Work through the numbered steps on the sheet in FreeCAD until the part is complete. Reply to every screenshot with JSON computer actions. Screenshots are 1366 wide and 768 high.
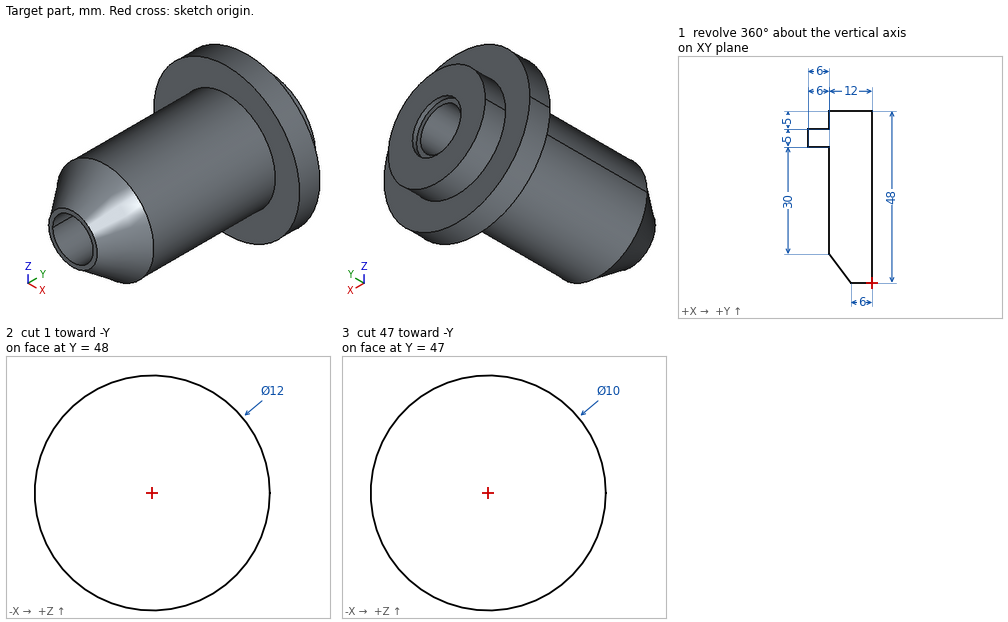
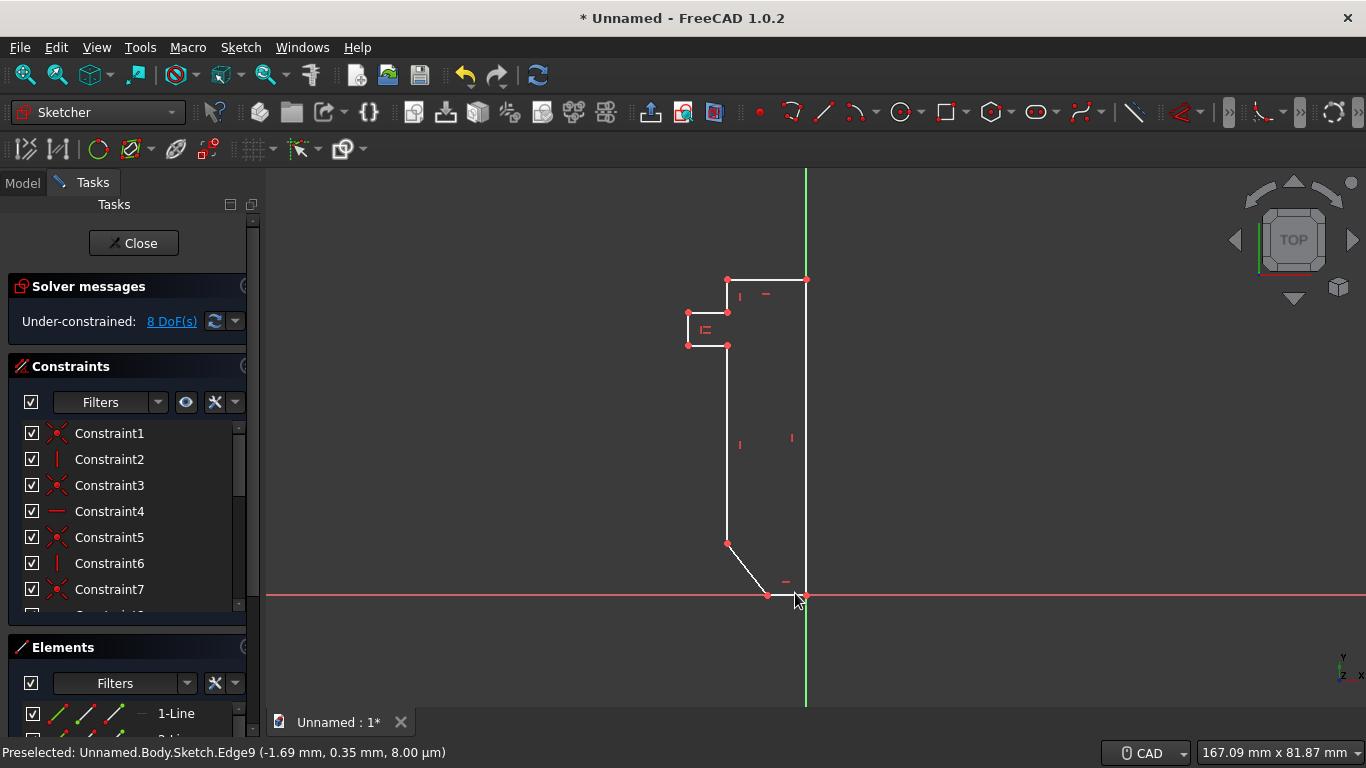
{"action": "scroll", "coordinate": [727, 290], "scroll_direction": "up", "scroll_amount": 2}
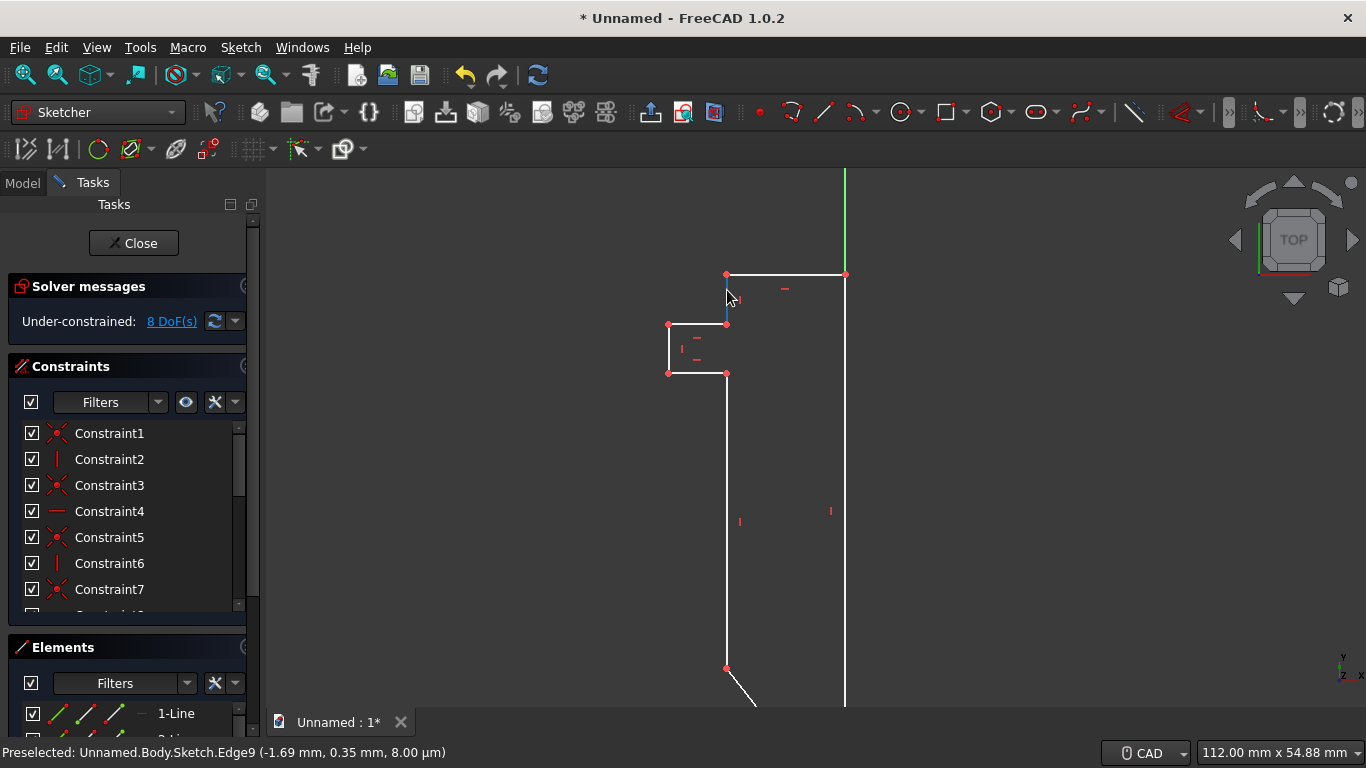
{"action": "left_click", "coordinate": [727, 290]}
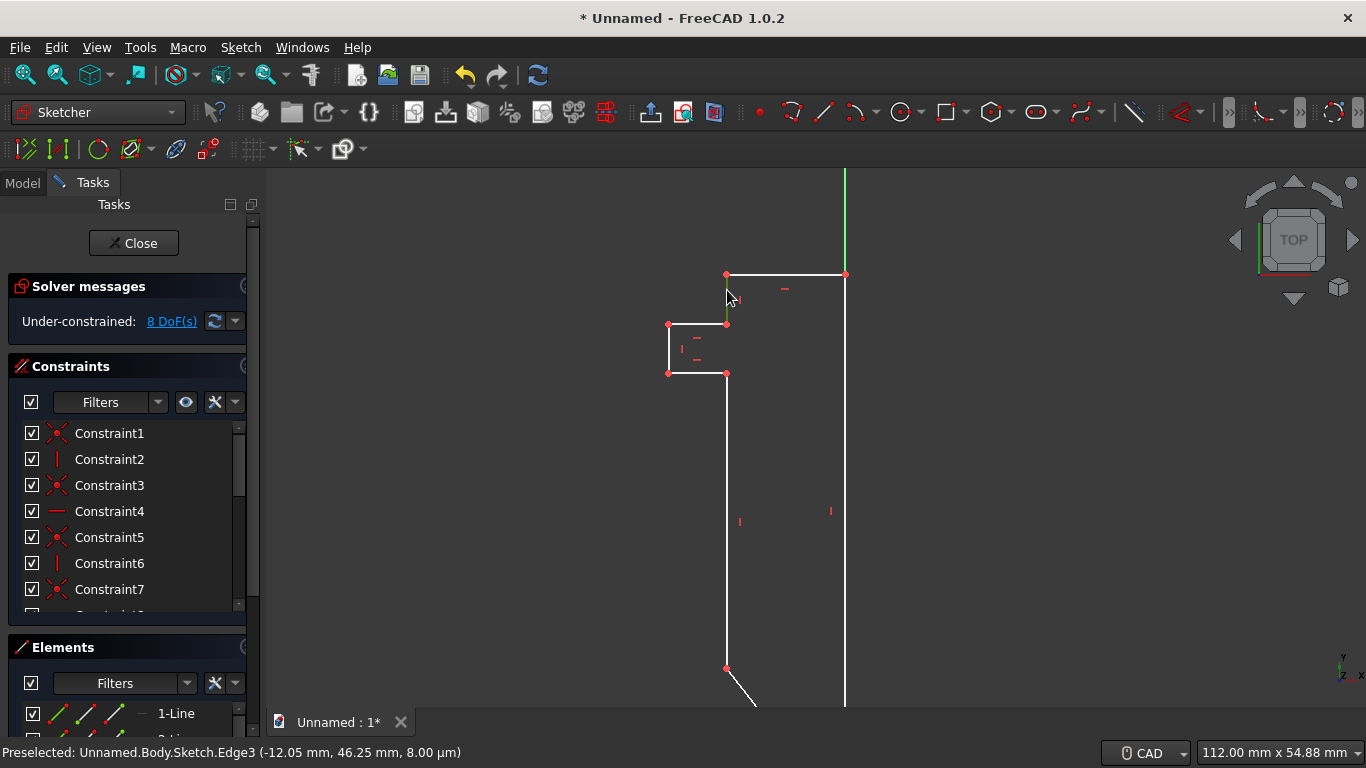
{"action": "left_click", "coordinate": [1202, 112]}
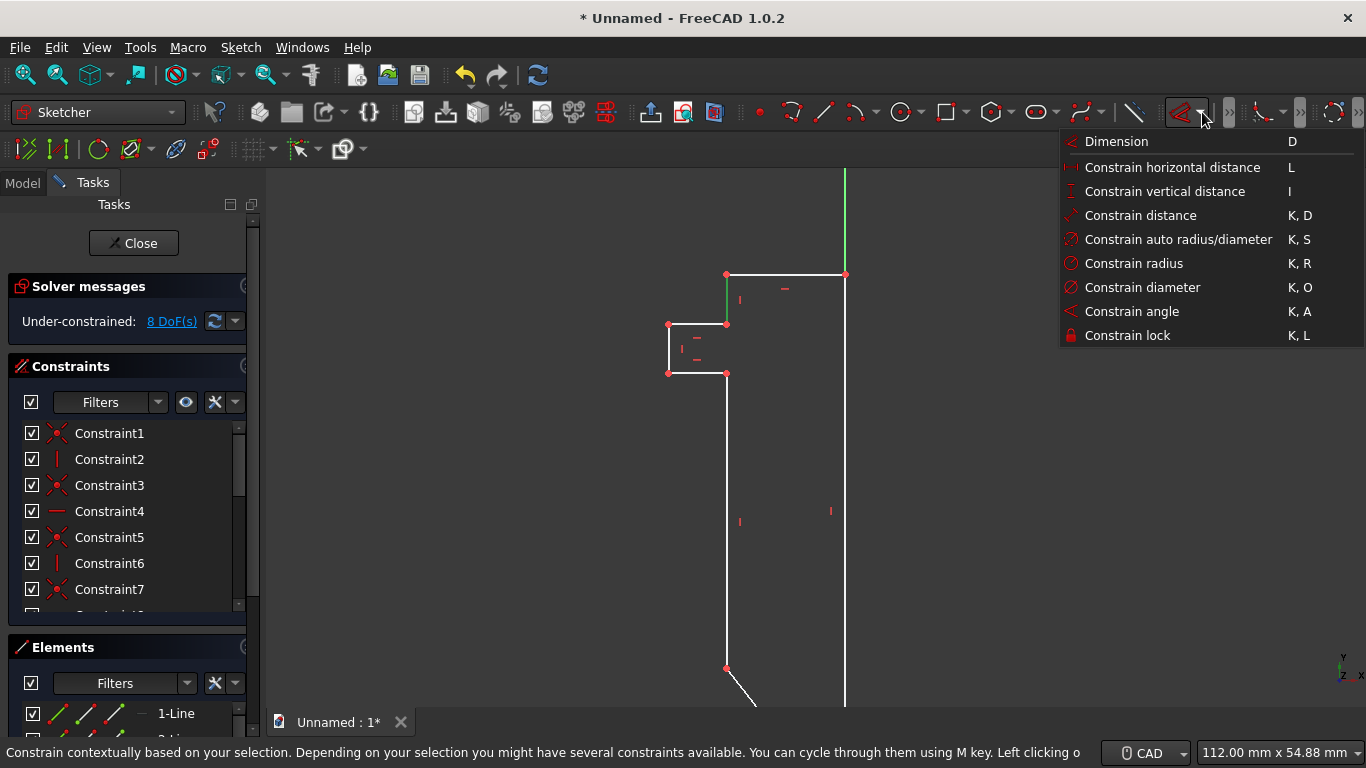
{"action": "left_click", "coordinate": [1212, 191]}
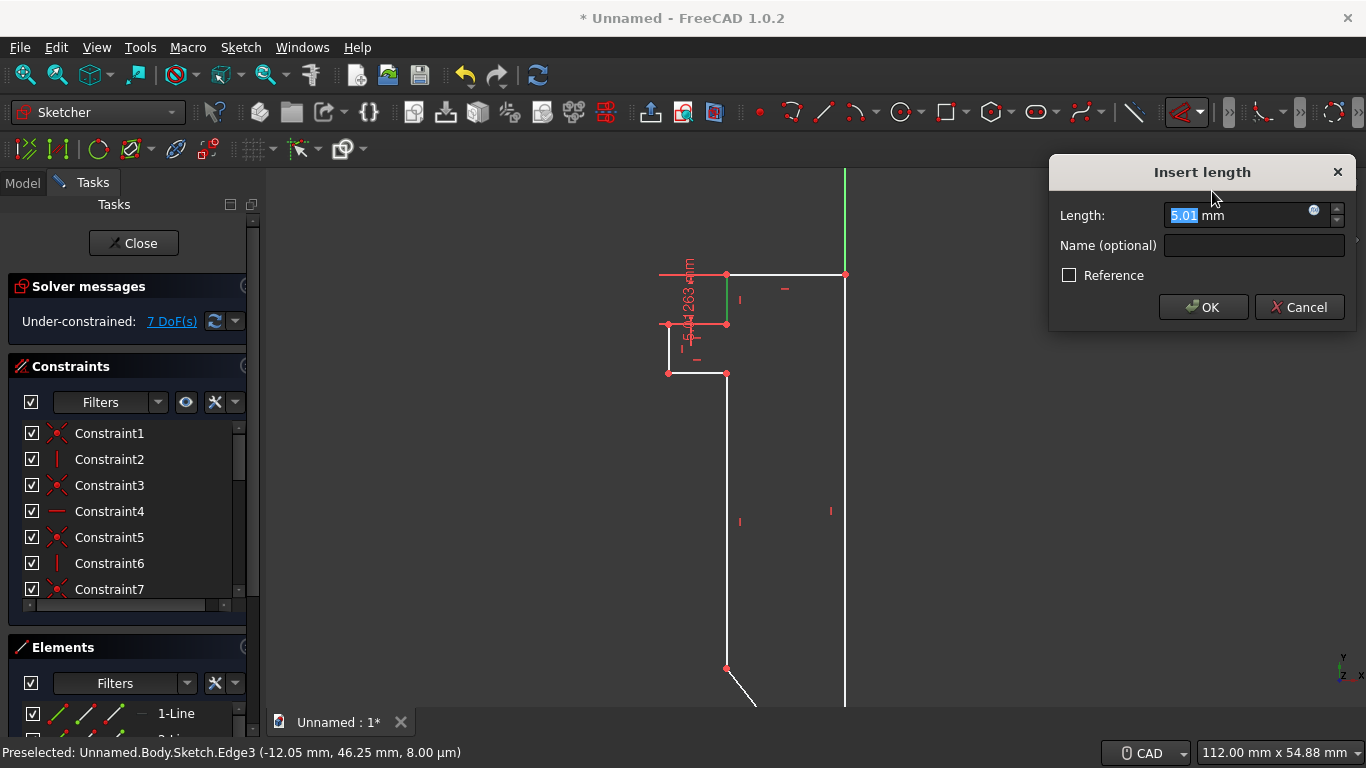
{"action": "type", "text": "5"}
{"action": "key", "text": "Return"}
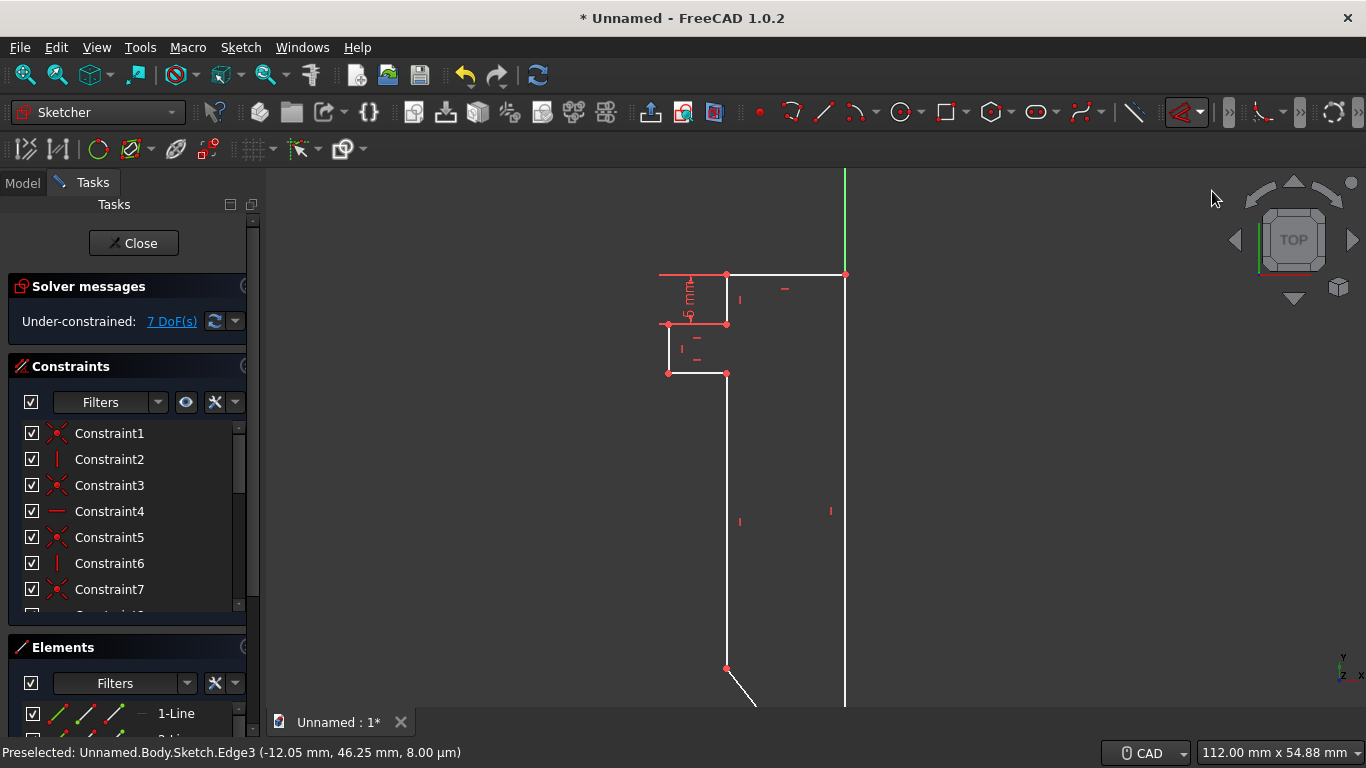
{"action": "left_click", "coordinate": [709, 324]}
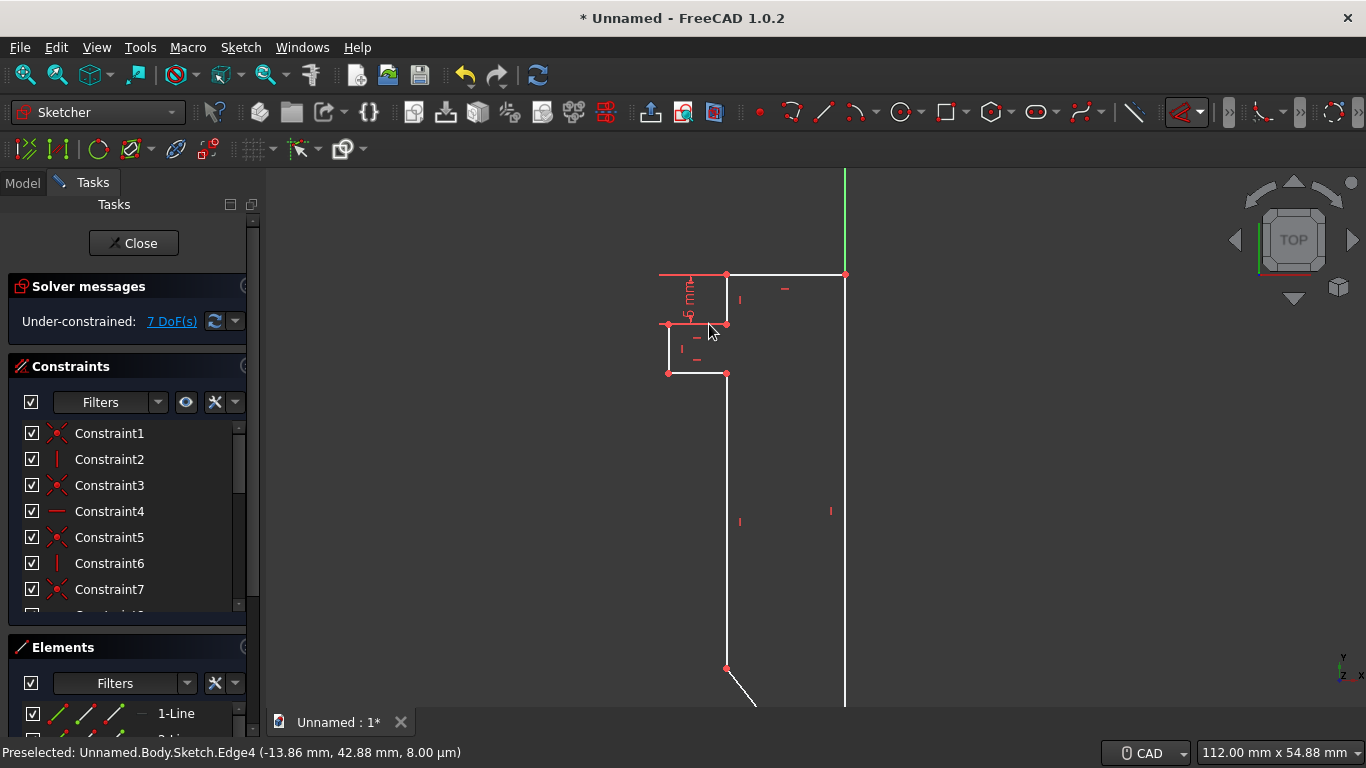
{"action": "left_click", "coordinate": [1202, 112]}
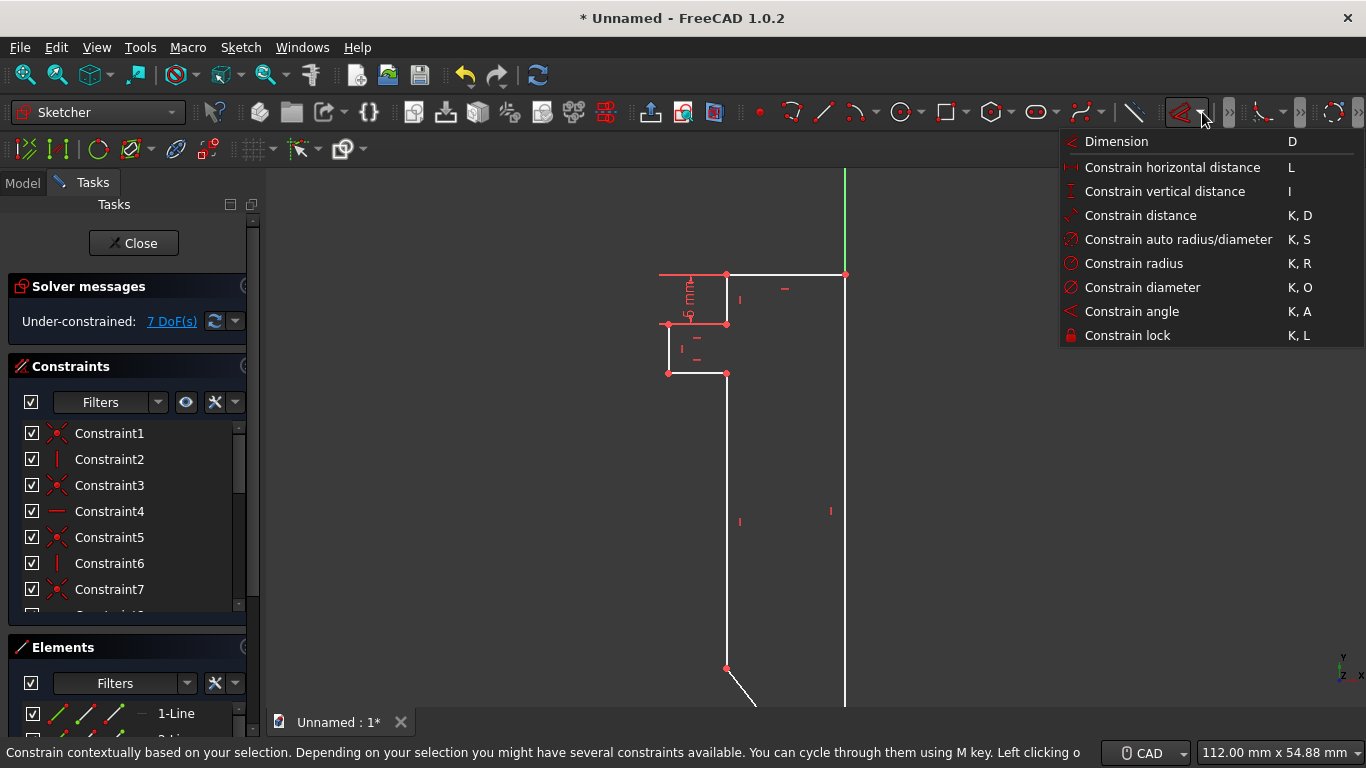
{"action": "left_click", "coordinate": [1212, 167]}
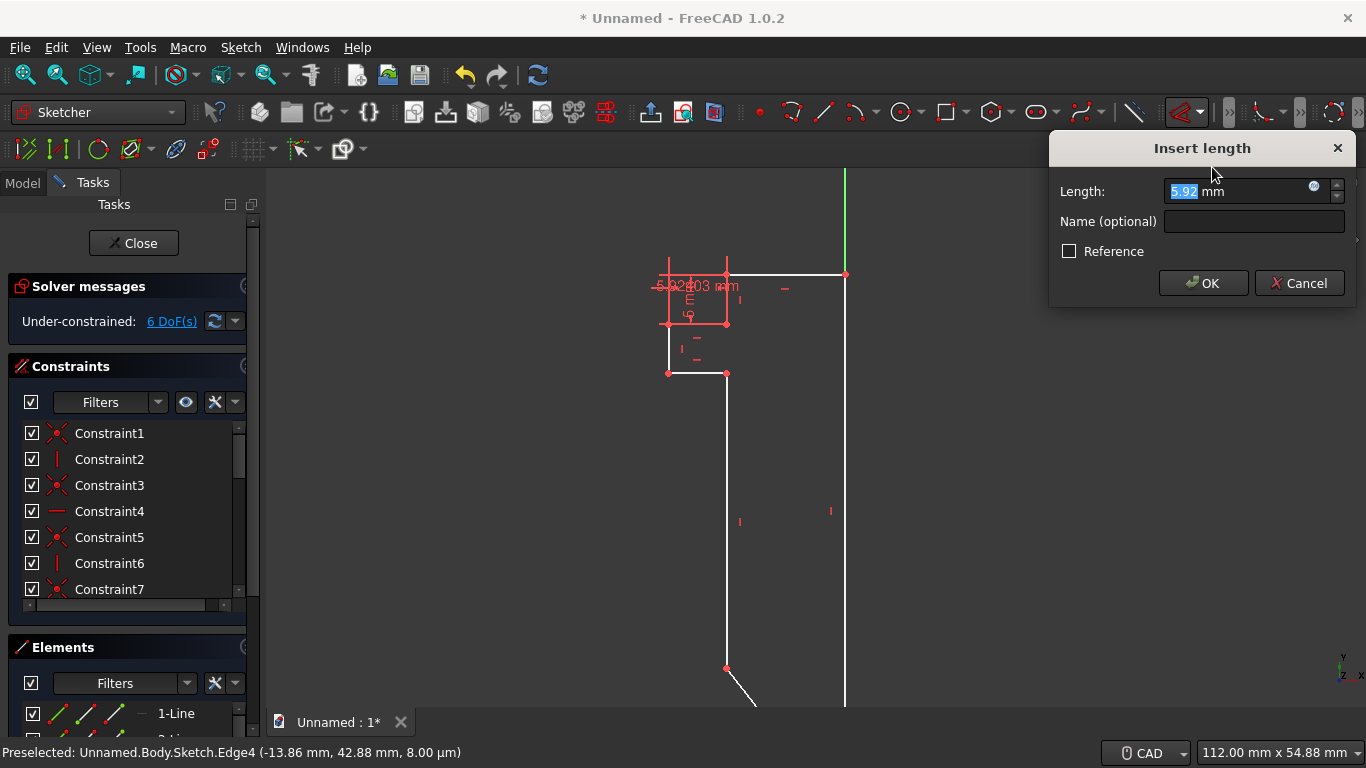
{"action": "type", "text": "6"}
{"action": "key", "text": "Return"}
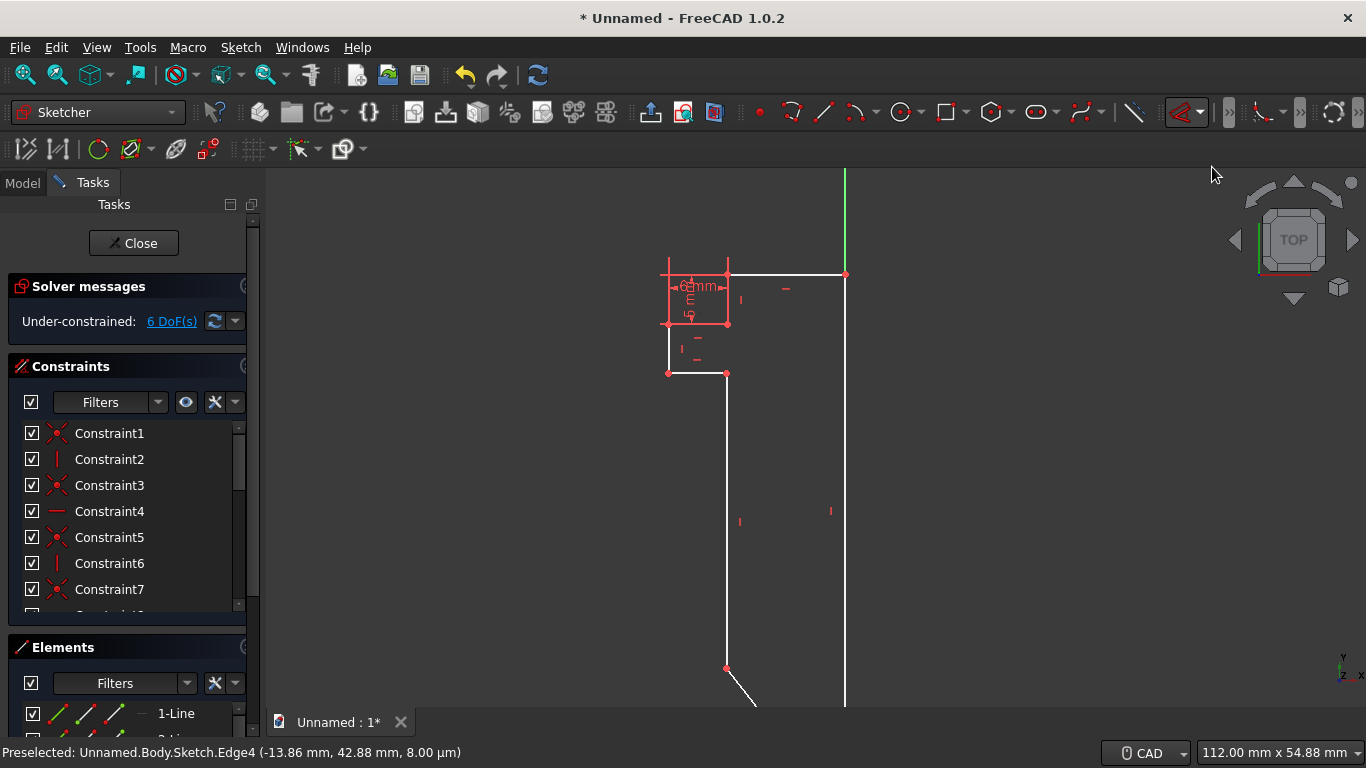
{"action": "left_click", "coordinate": [669, 339]}